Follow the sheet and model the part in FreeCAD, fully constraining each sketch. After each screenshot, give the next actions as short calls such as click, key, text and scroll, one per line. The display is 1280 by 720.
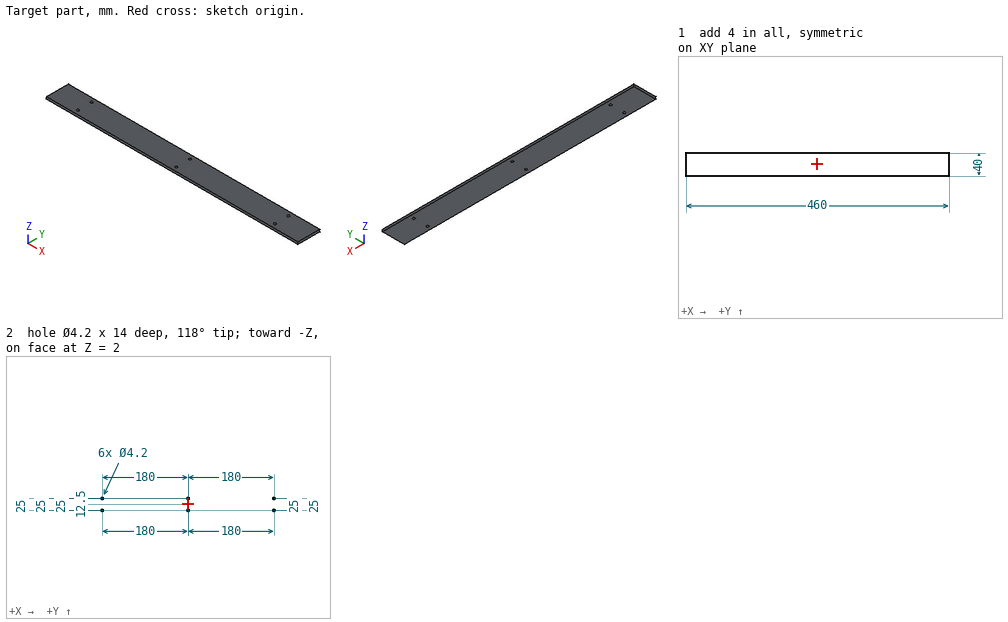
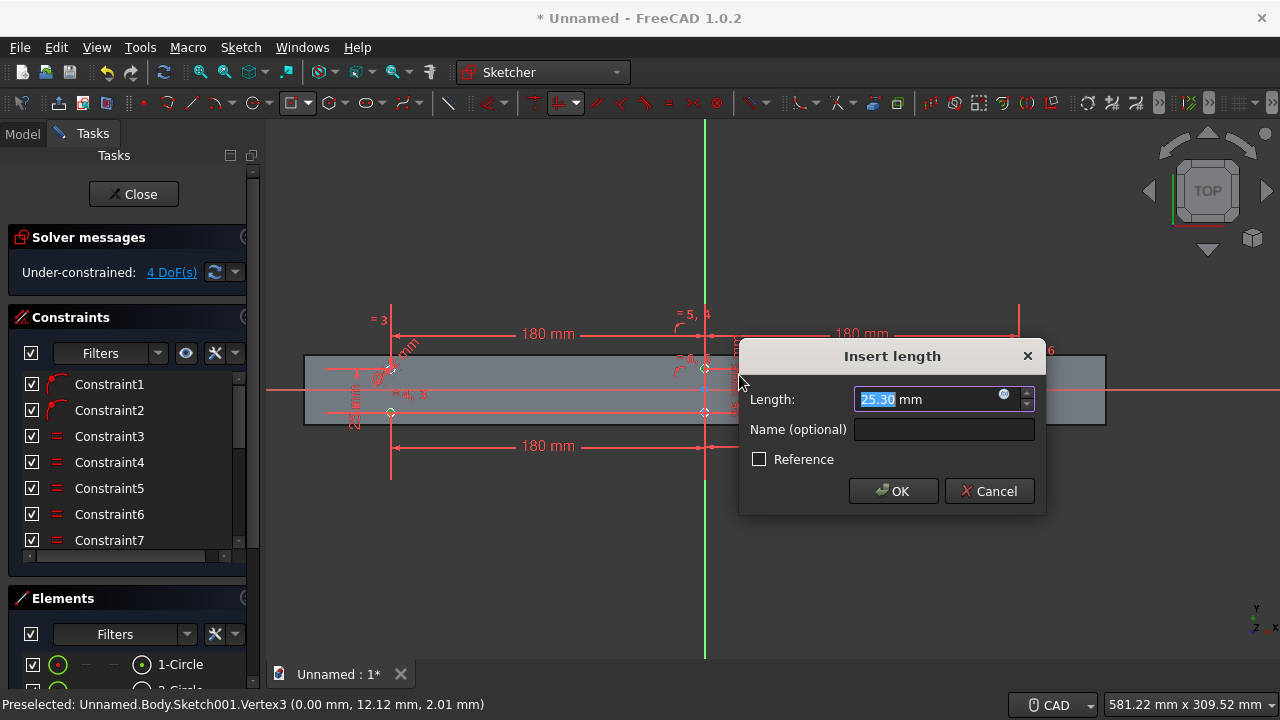
text(25)
key(Return)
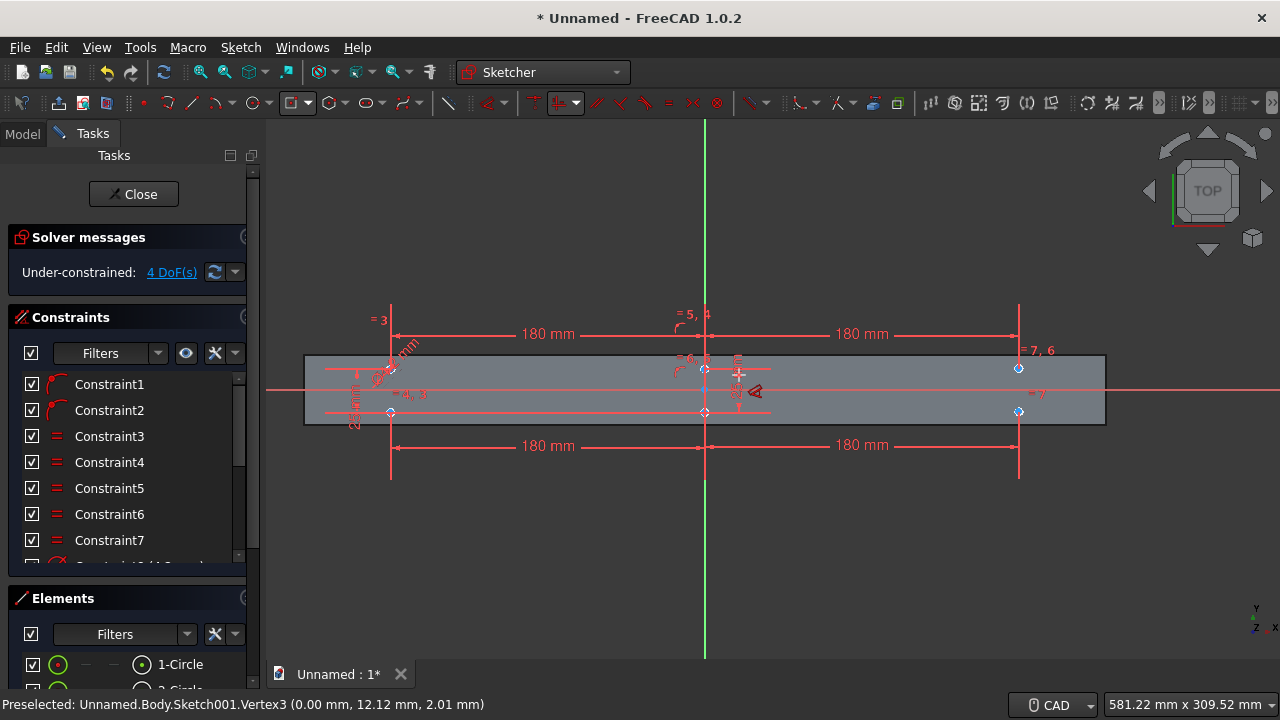
click(705, 369)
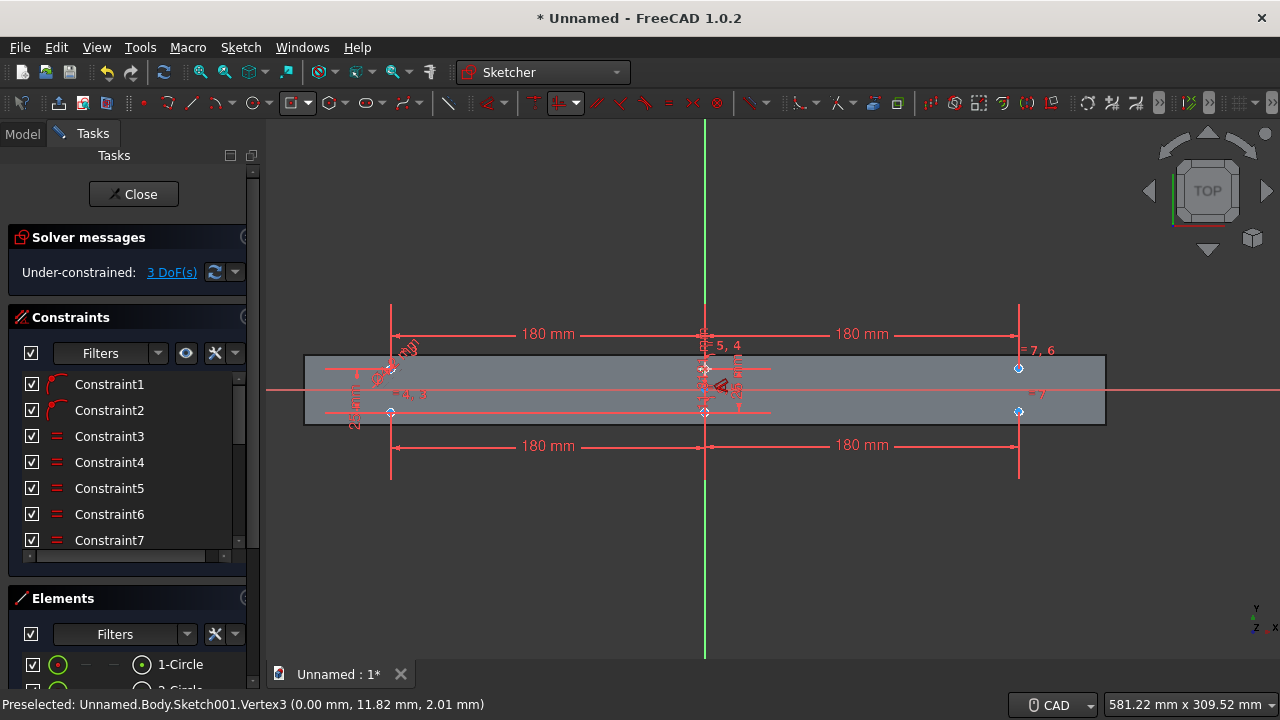
click(705, 413)
click(739, 406)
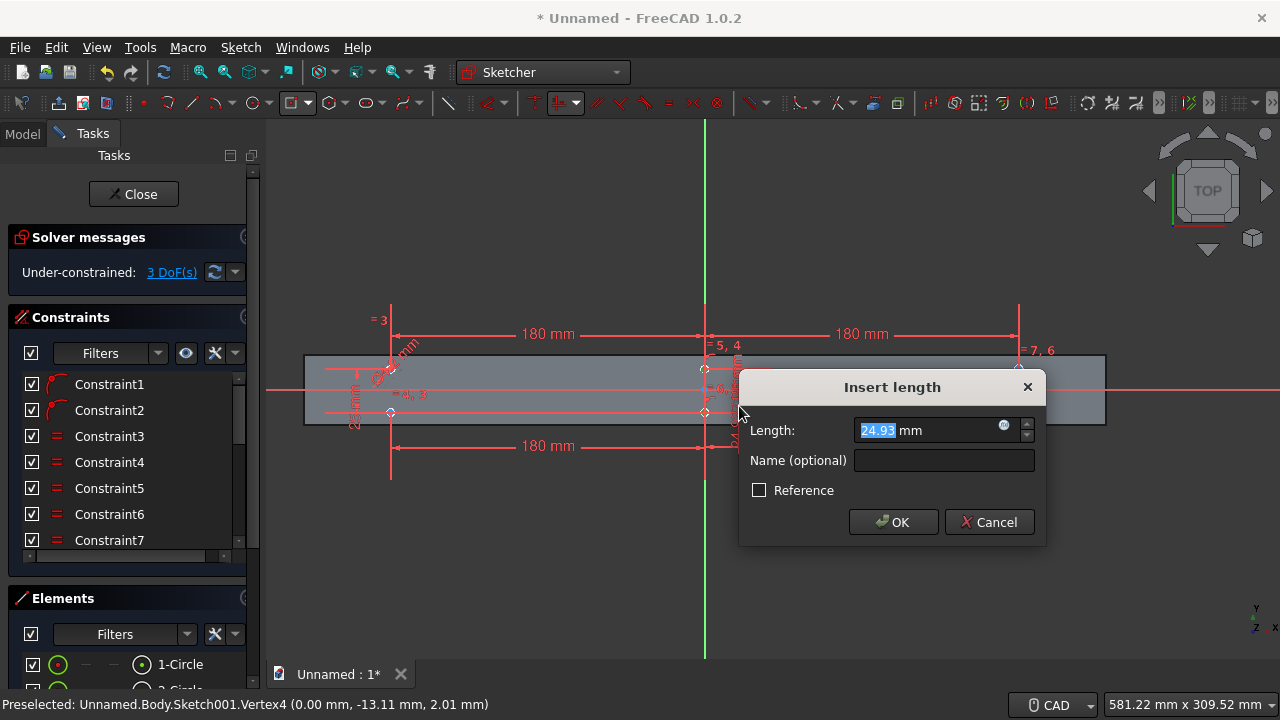
text(25)
key(Return)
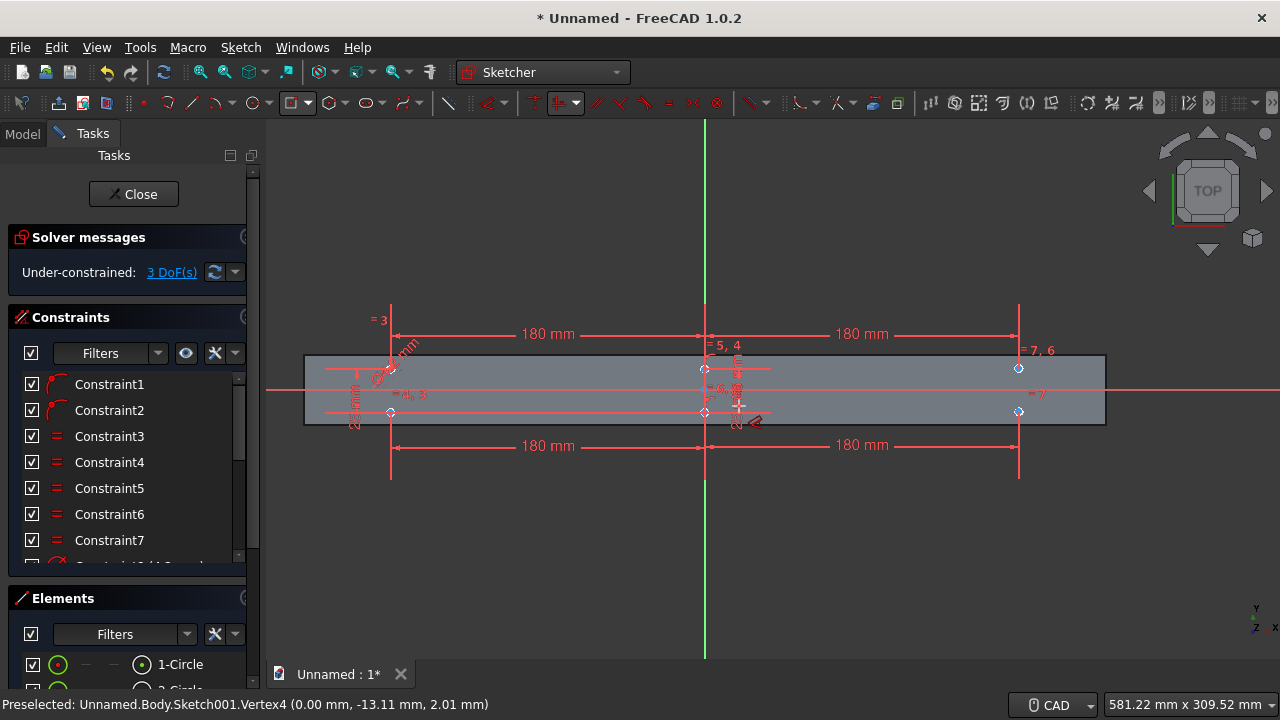
click(705, 413)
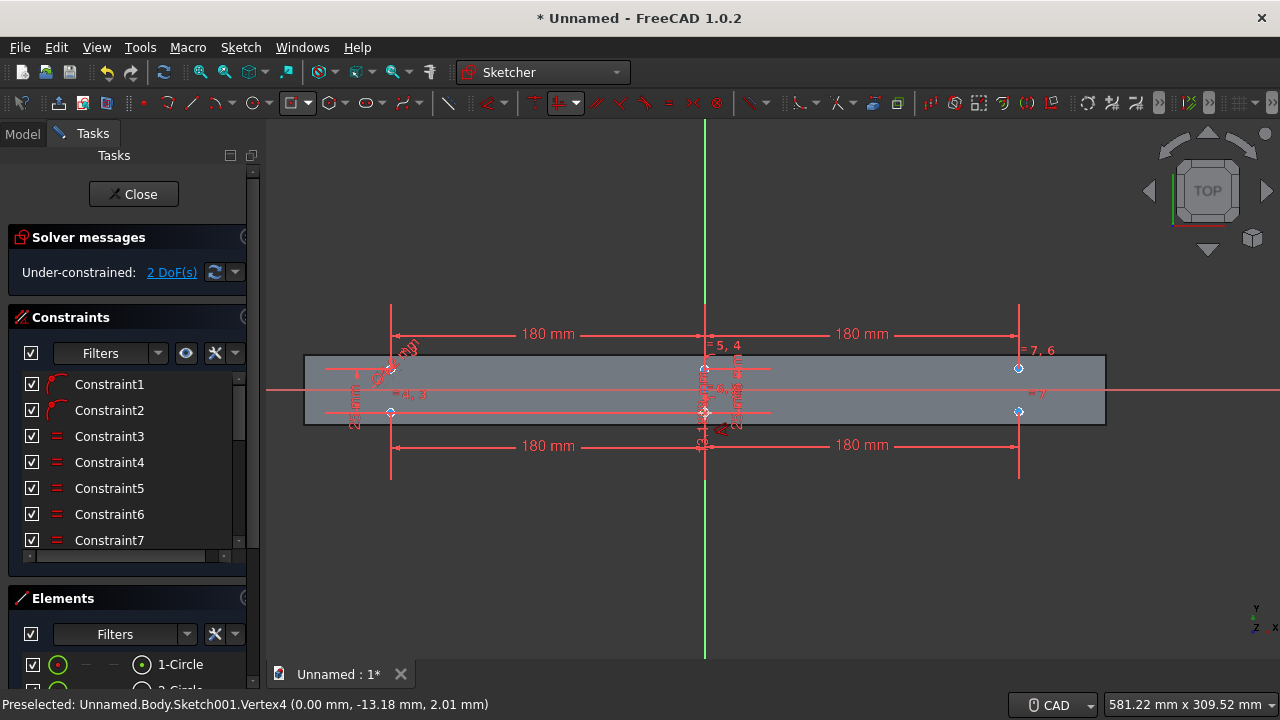
click(1019, 369)
click(1053, 375)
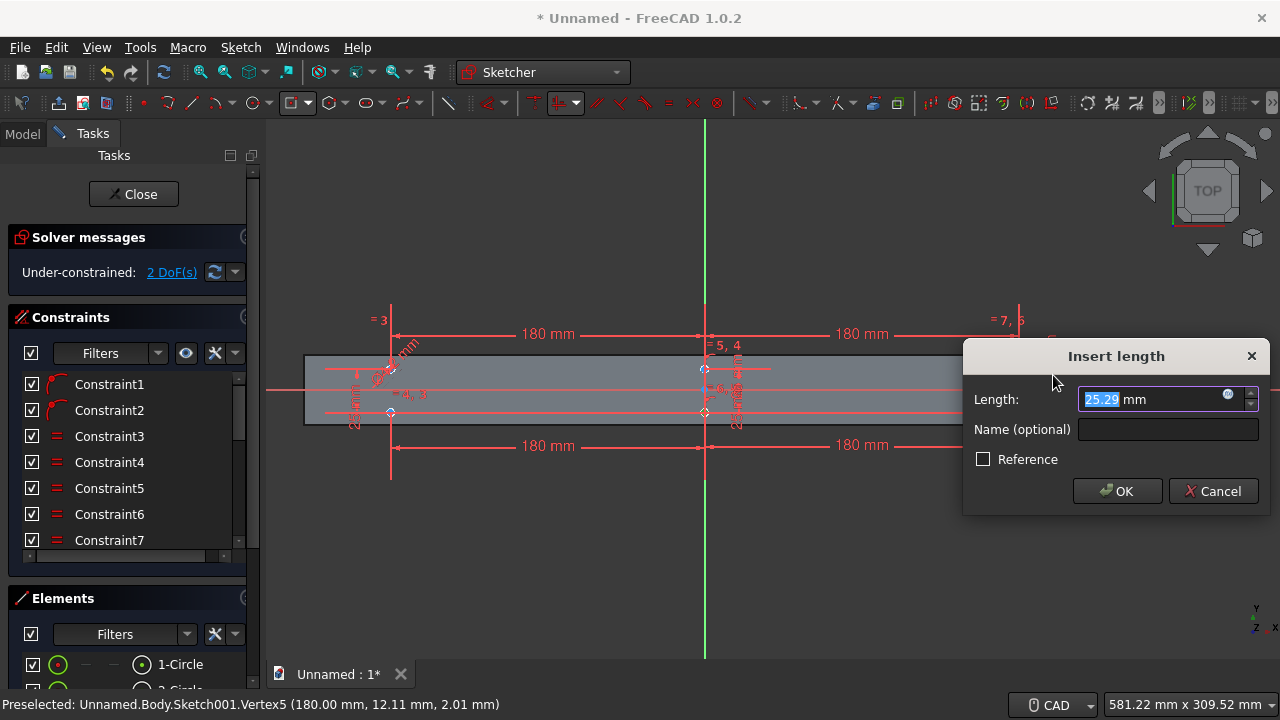
text(25)
key(Return)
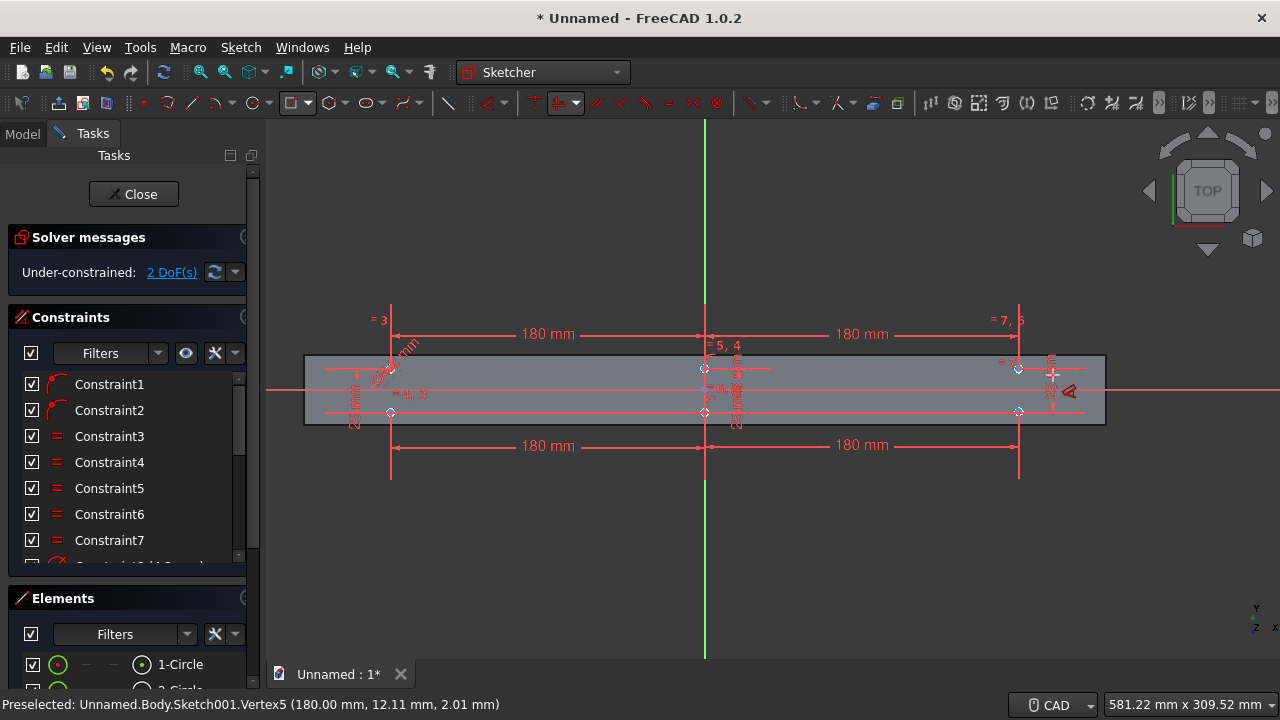
click(1019, 369)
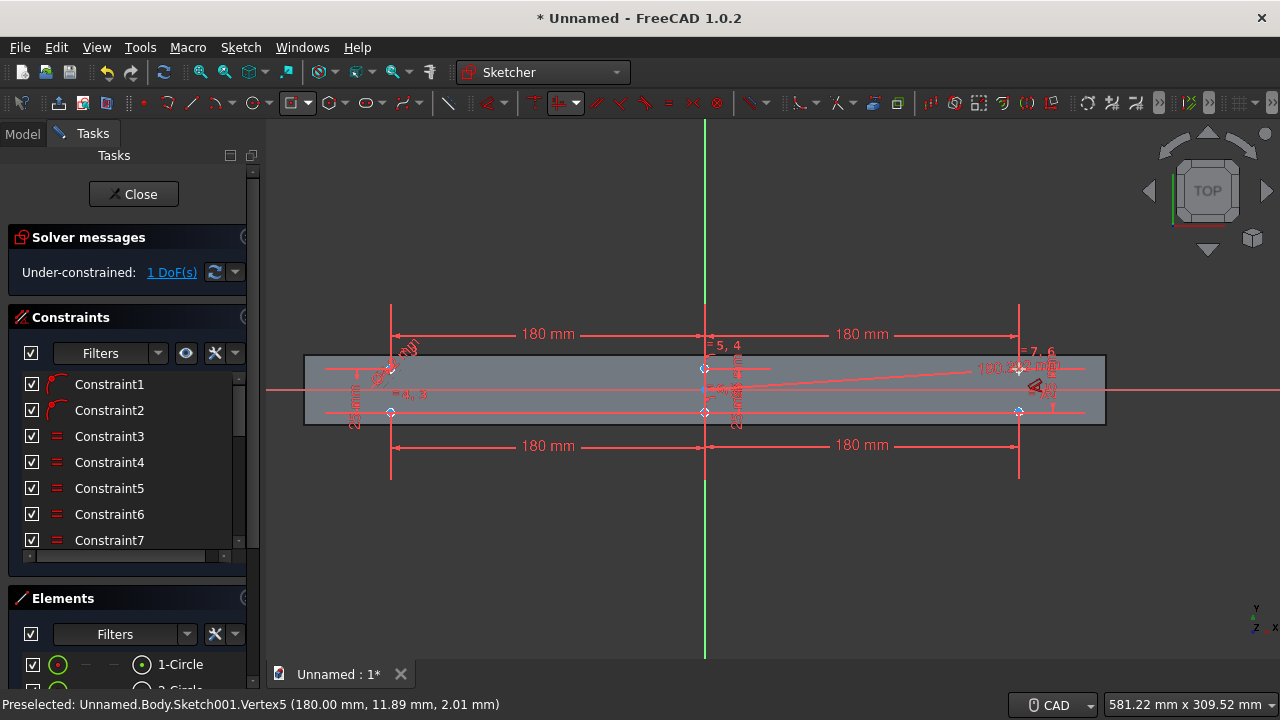
click(1019, 412)
click(1053, 406)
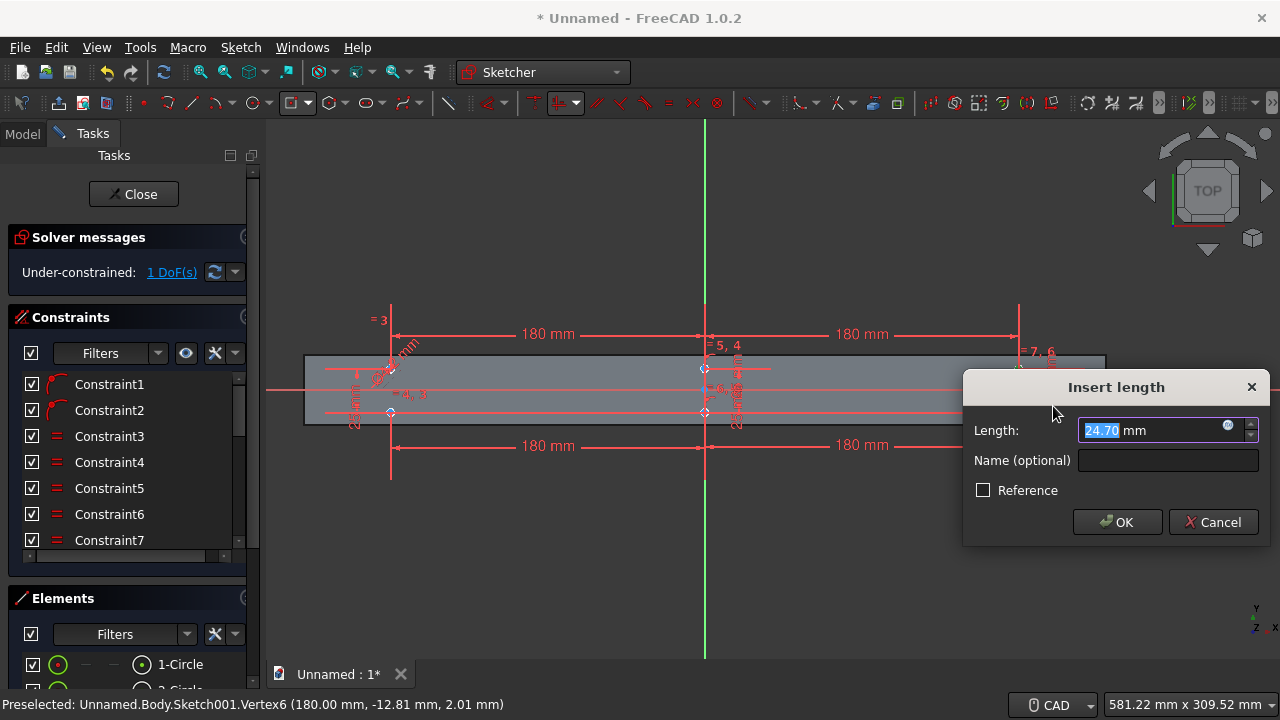
text(25)
key(Return)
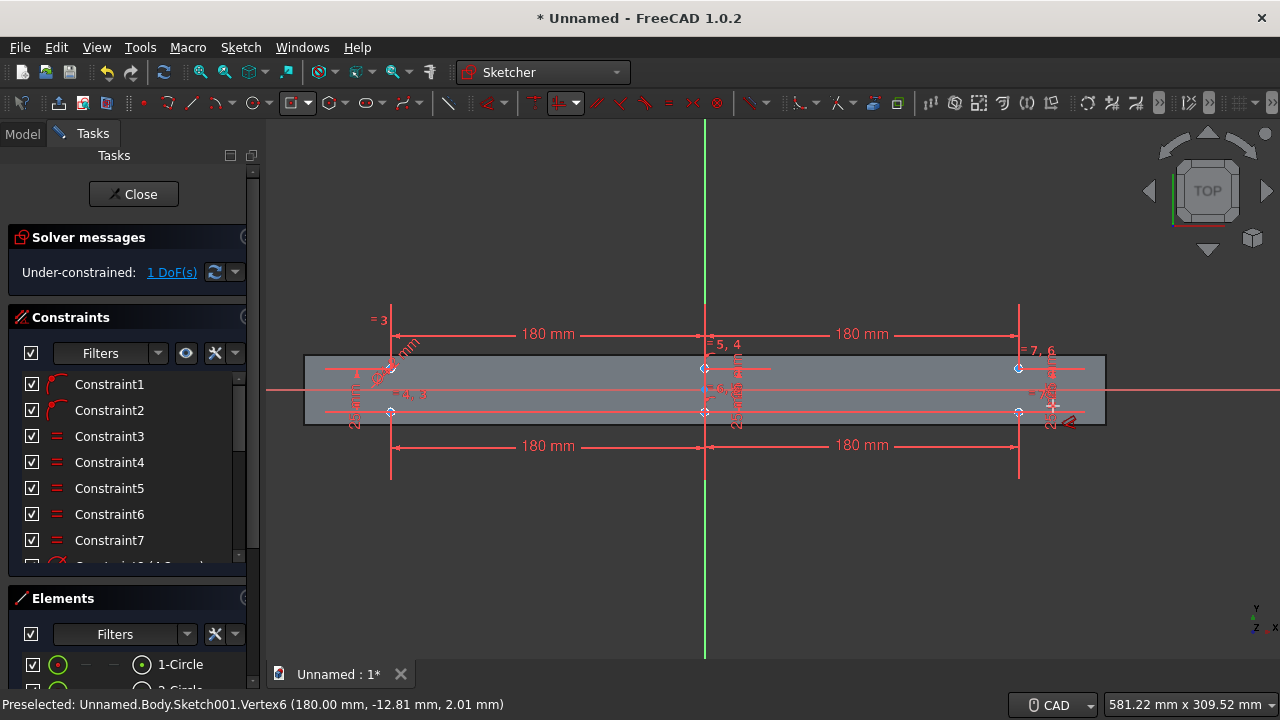
scroll(391, 369, up, 3)